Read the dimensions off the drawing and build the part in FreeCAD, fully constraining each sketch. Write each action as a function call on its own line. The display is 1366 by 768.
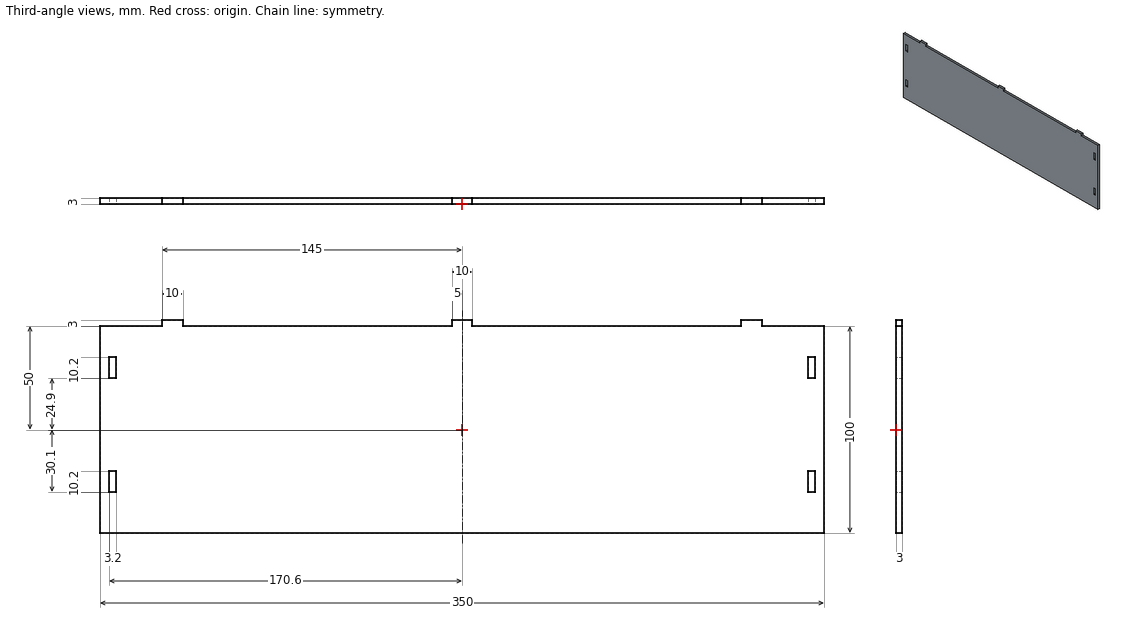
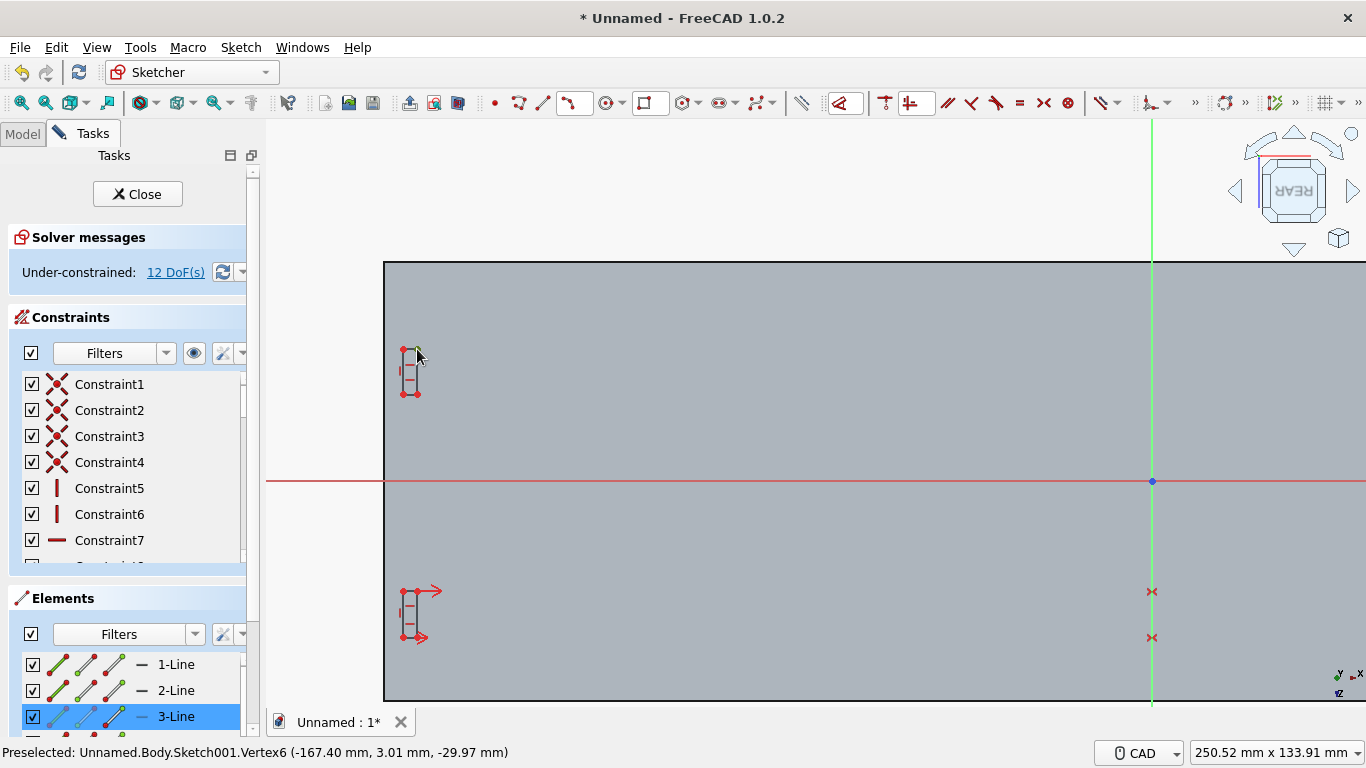
scroll(417, 348, down, 4)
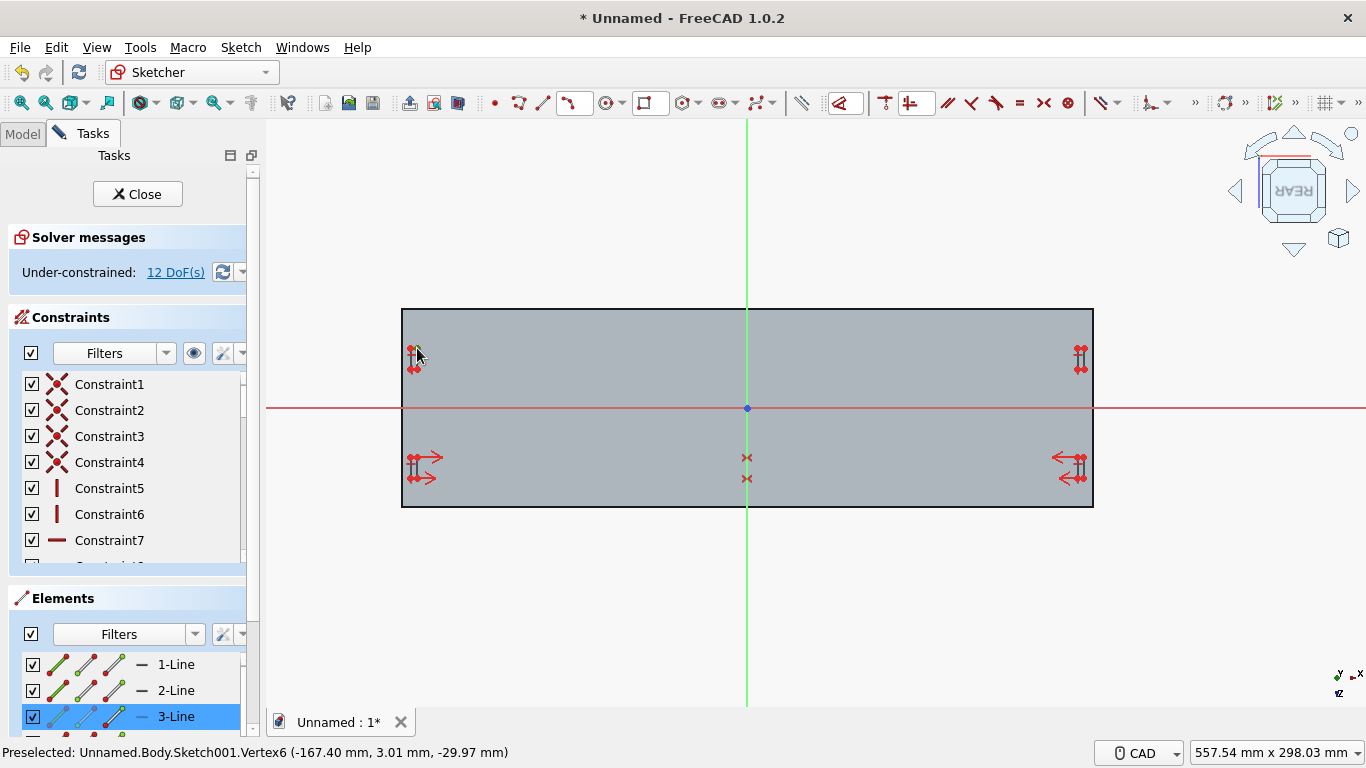
scroll(1078, 349, up, 4)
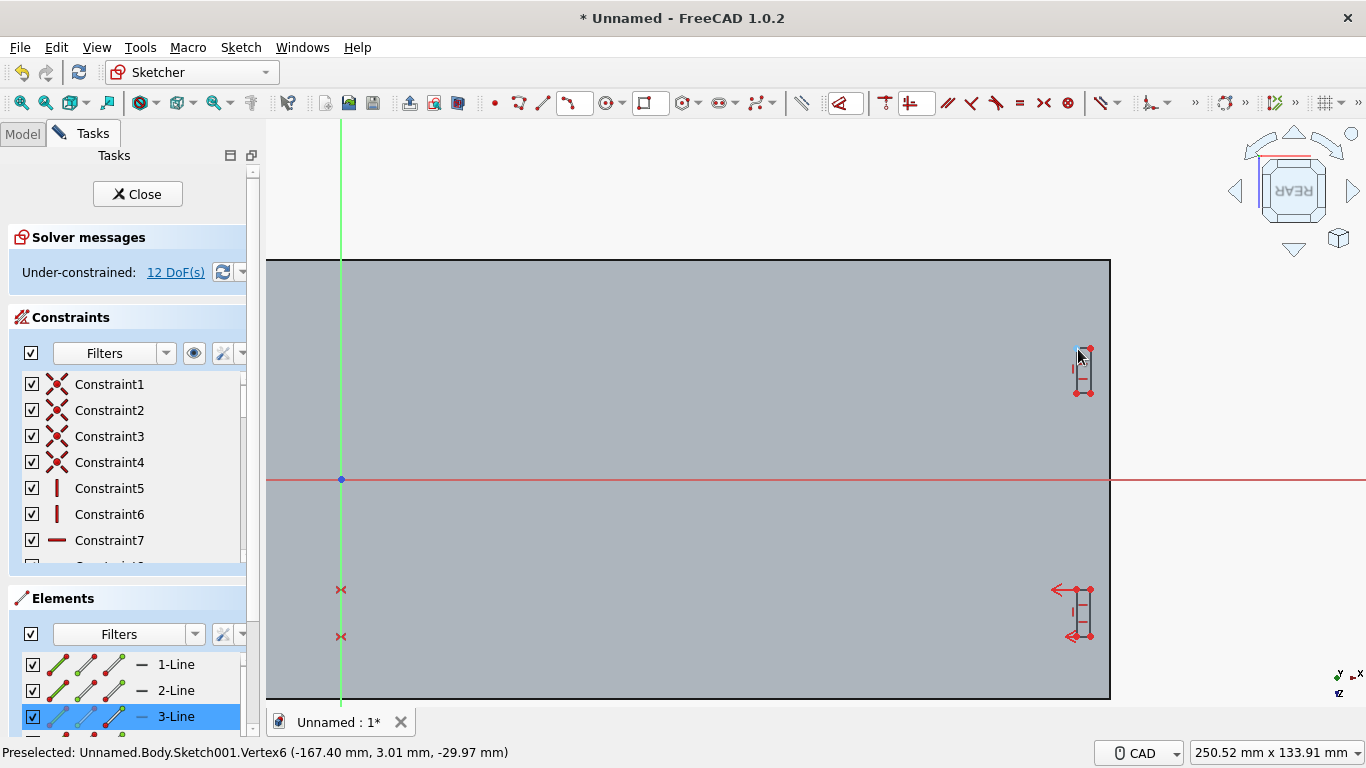
click(1077, 348)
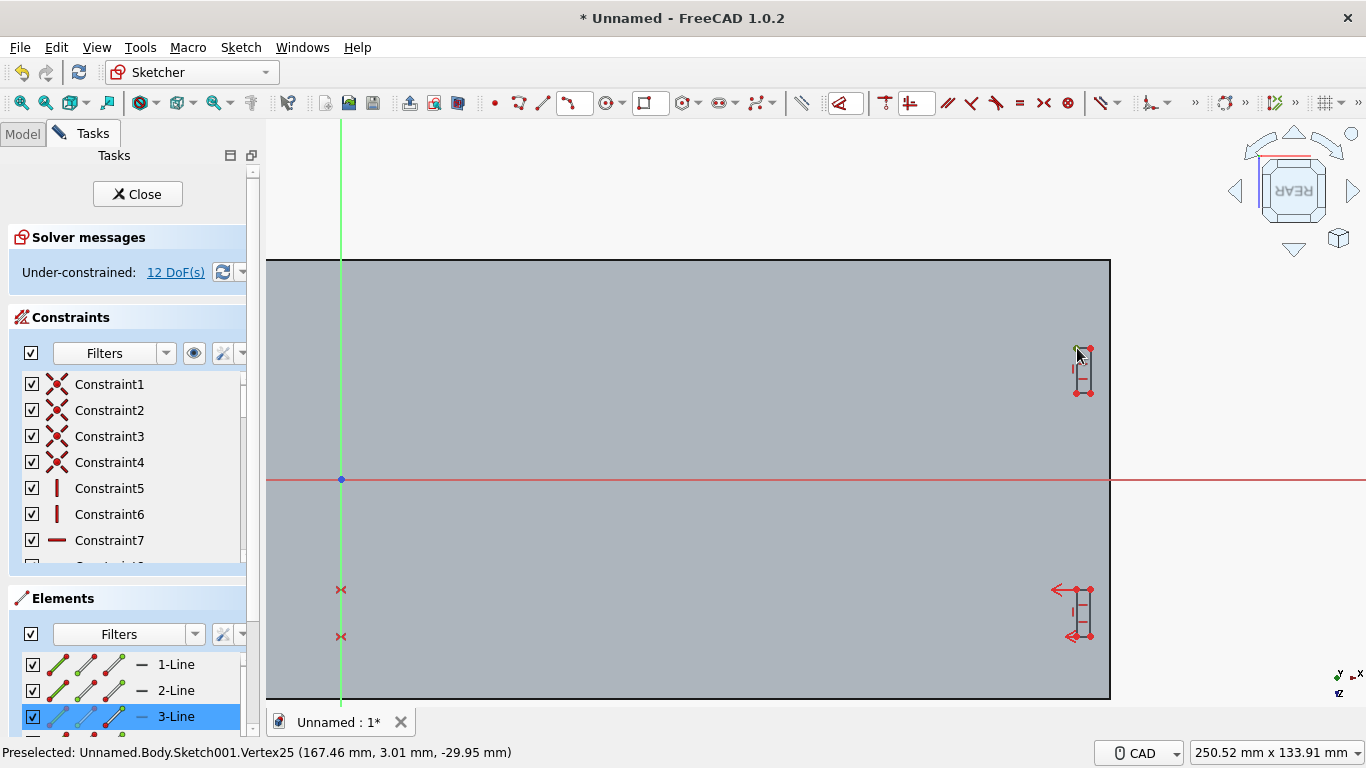
click(341, 603)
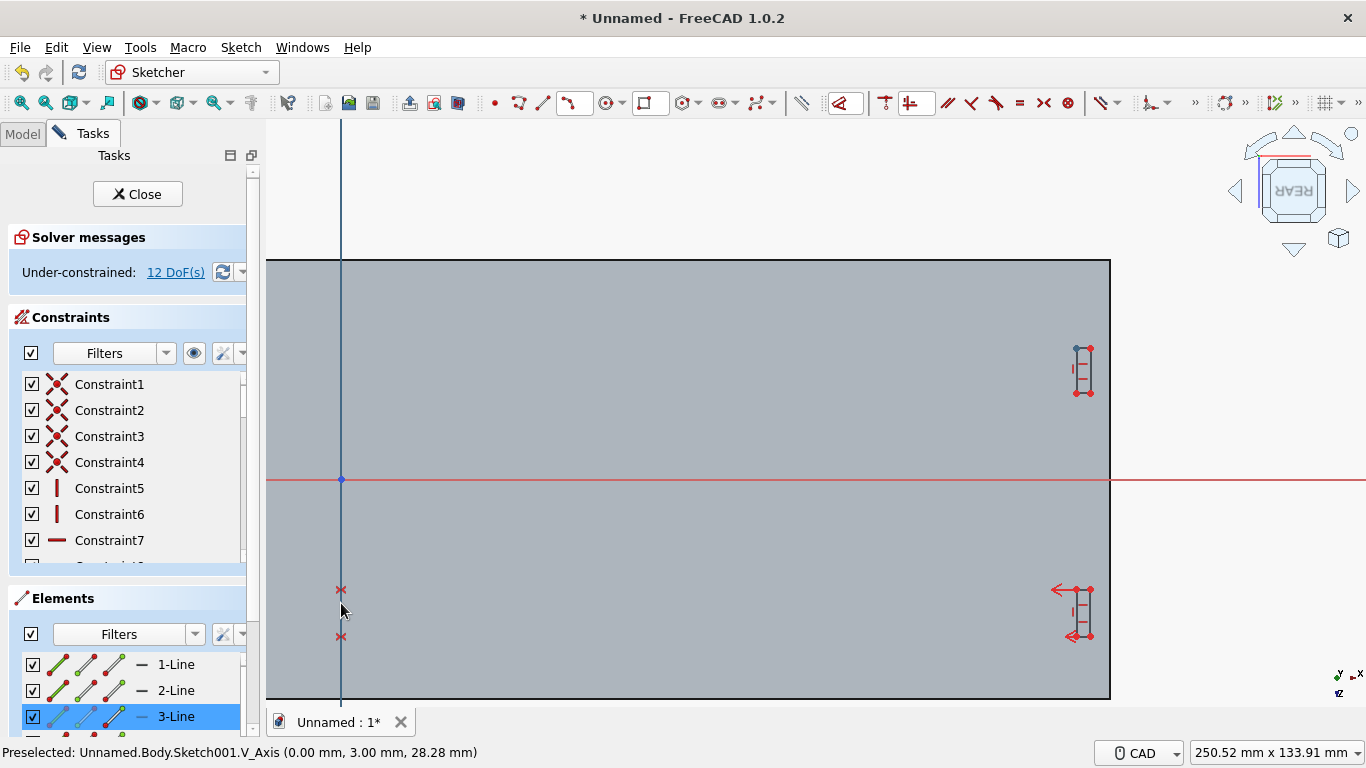
key(s)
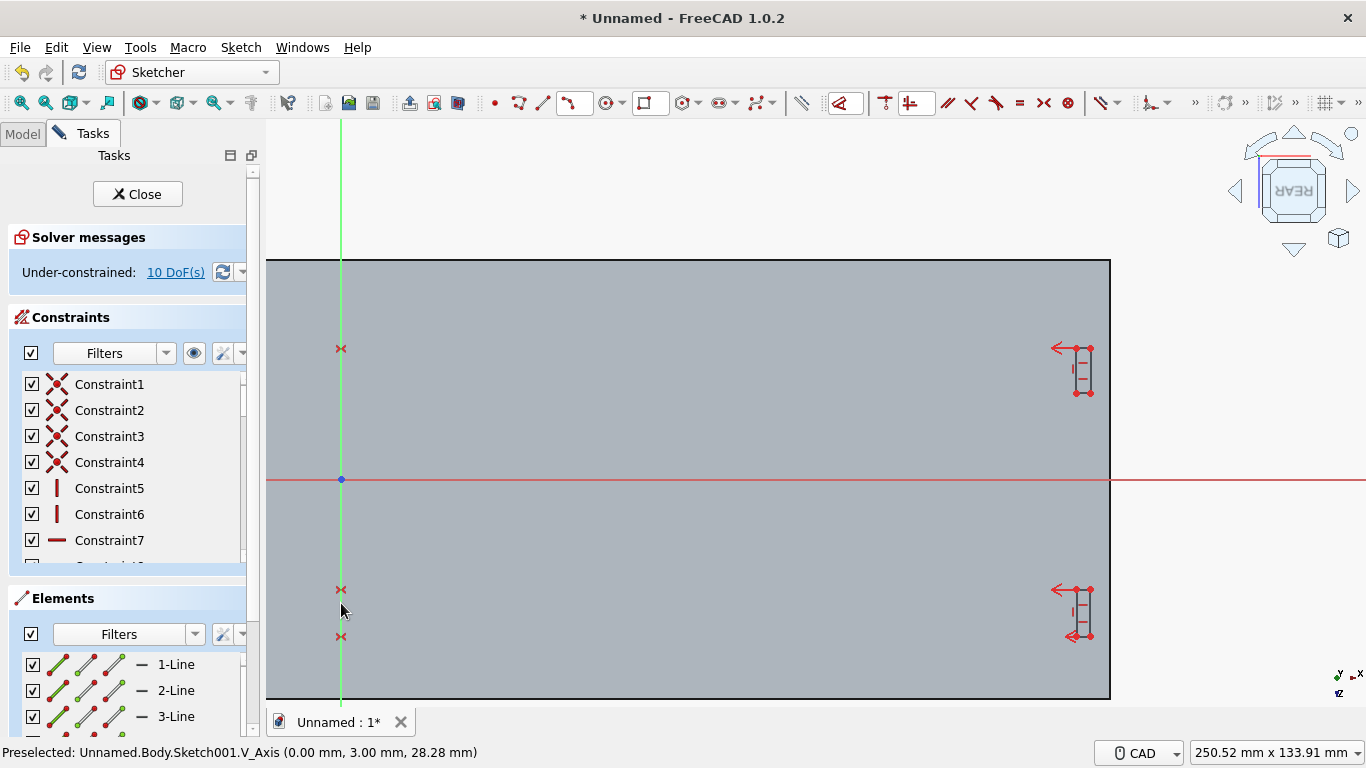
scroll(1079, 350, down, 4)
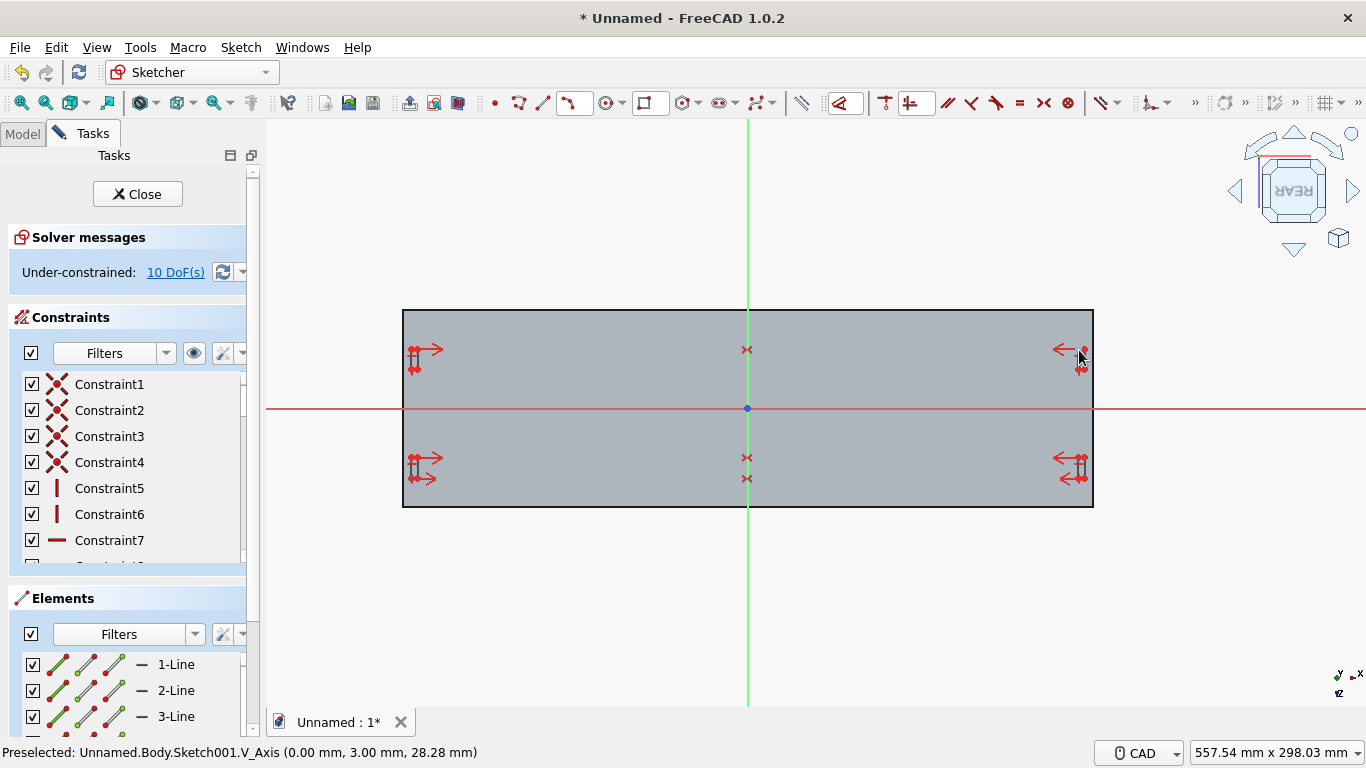
scroll(411, 370, up, 4)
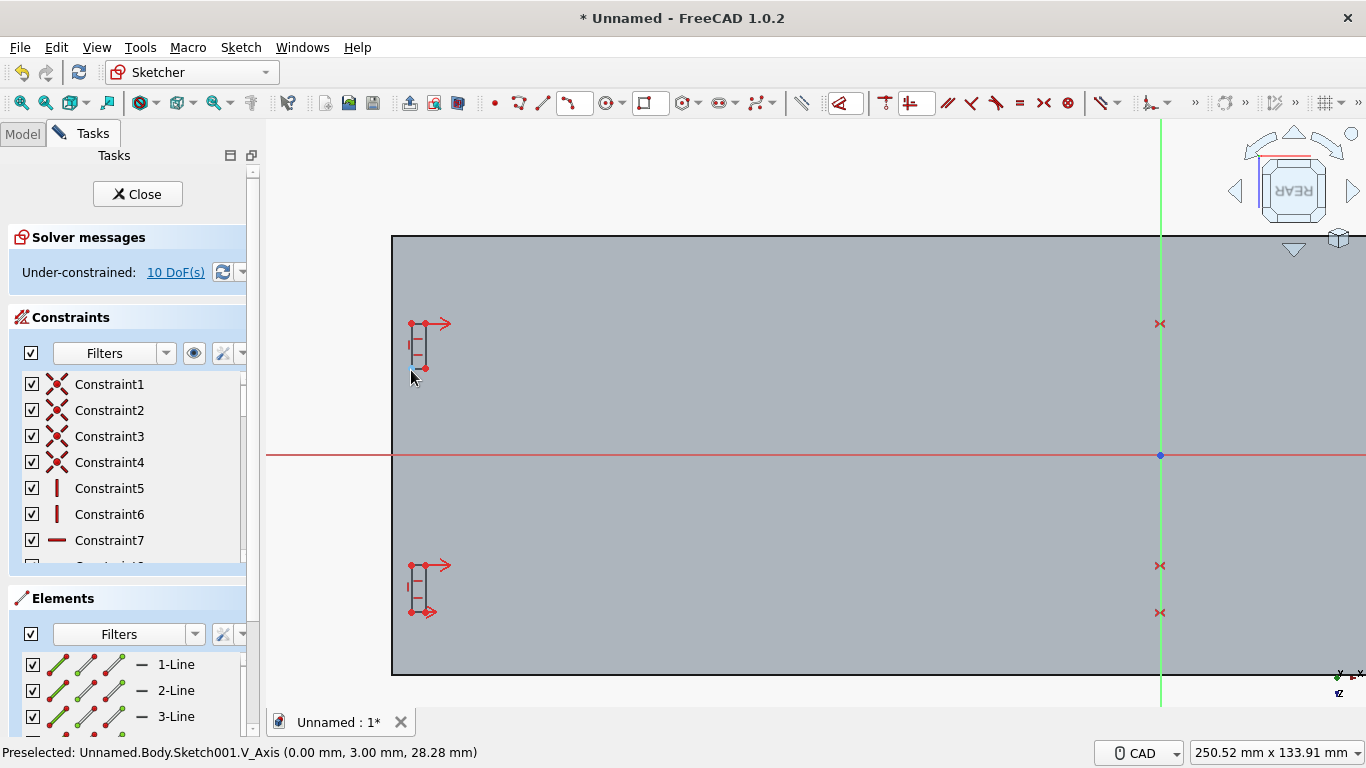
click(412, 369)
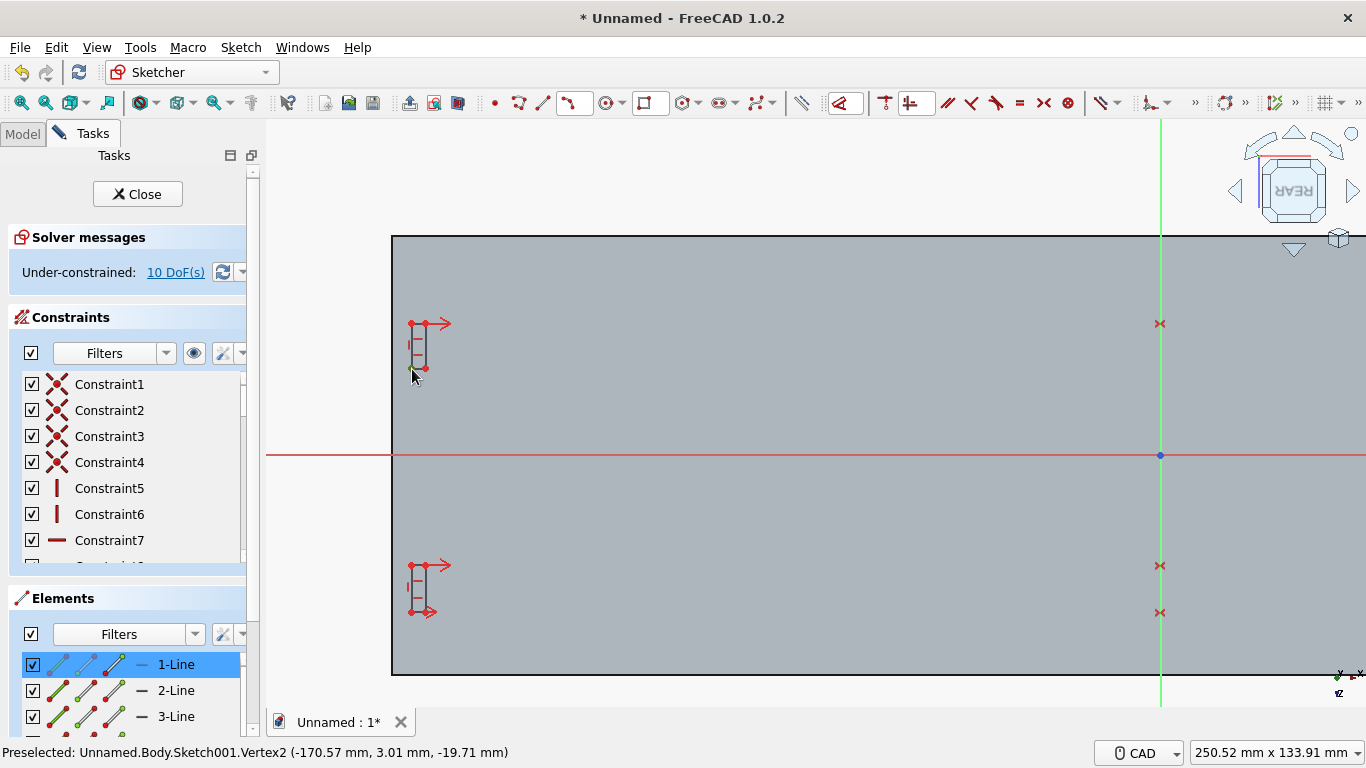
scroll(410, 370, down, 4)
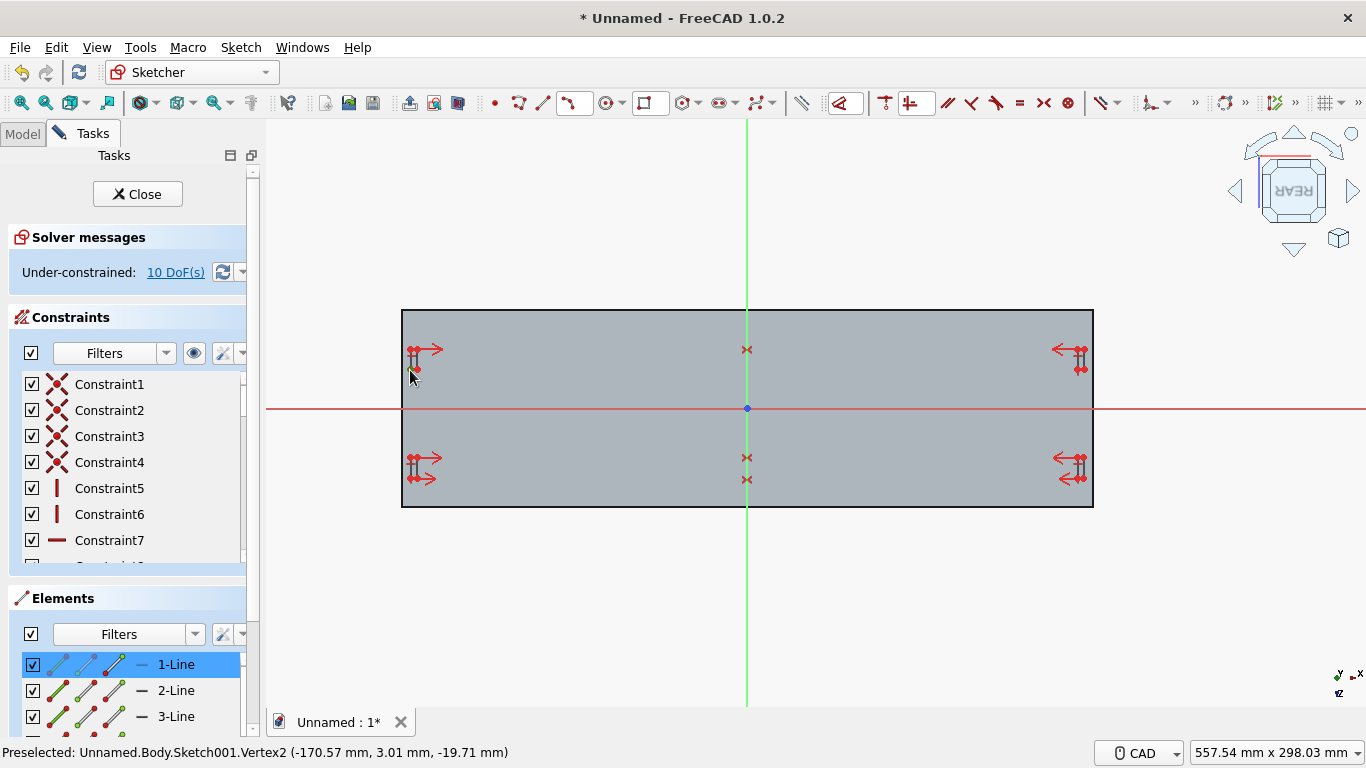
scroll(1084, 370, up, 4)